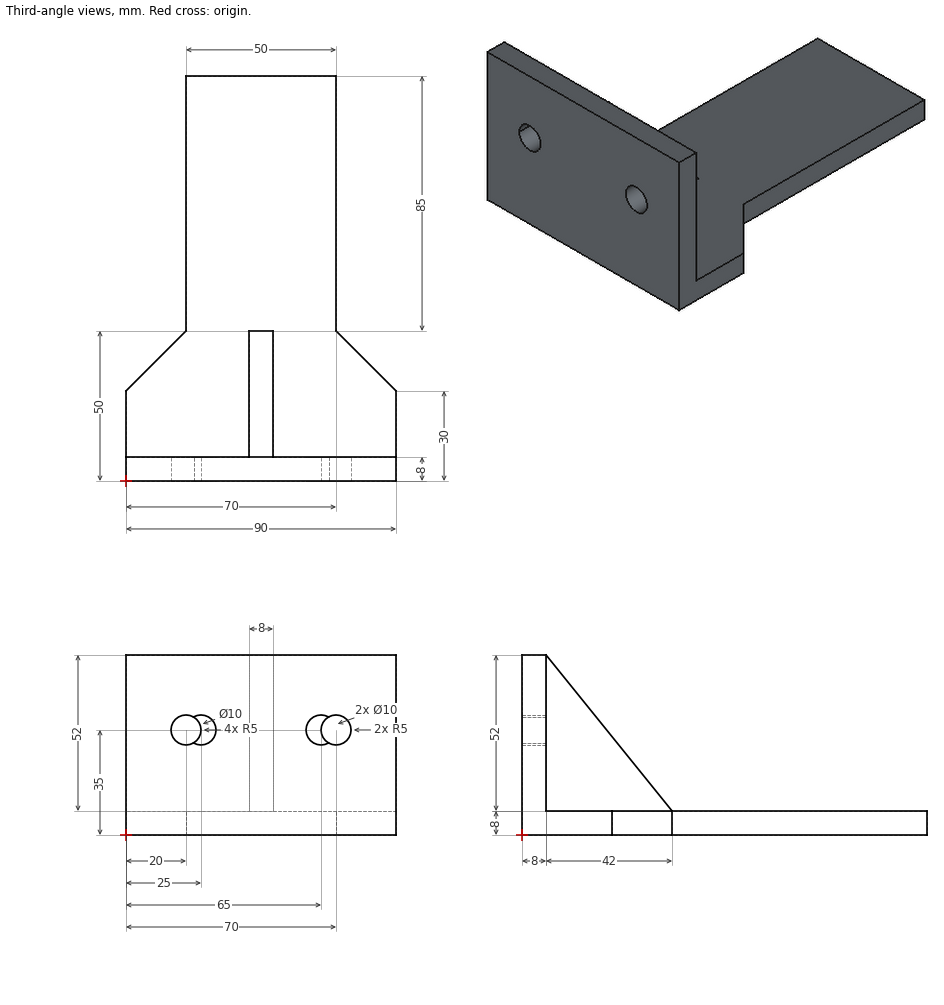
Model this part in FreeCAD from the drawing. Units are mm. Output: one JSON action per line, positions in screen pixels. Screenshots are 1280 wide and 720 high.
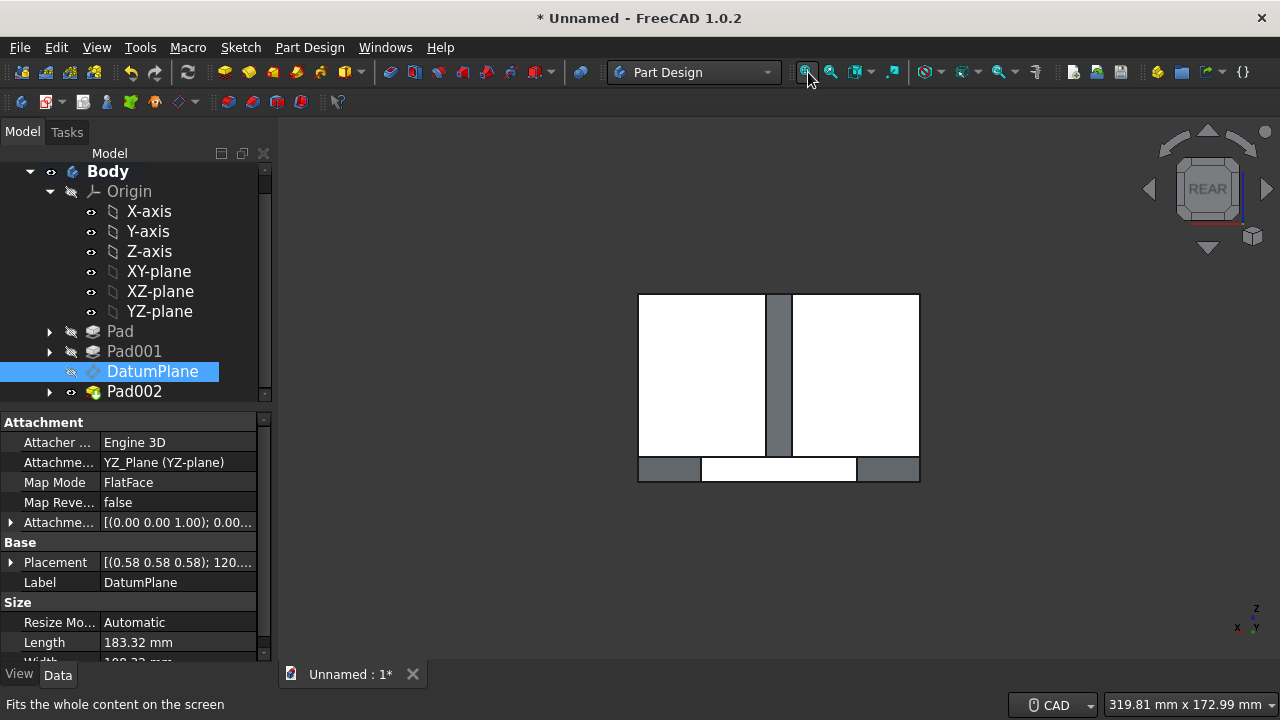
{"action": "left_click", "coordinate": [856, 374]}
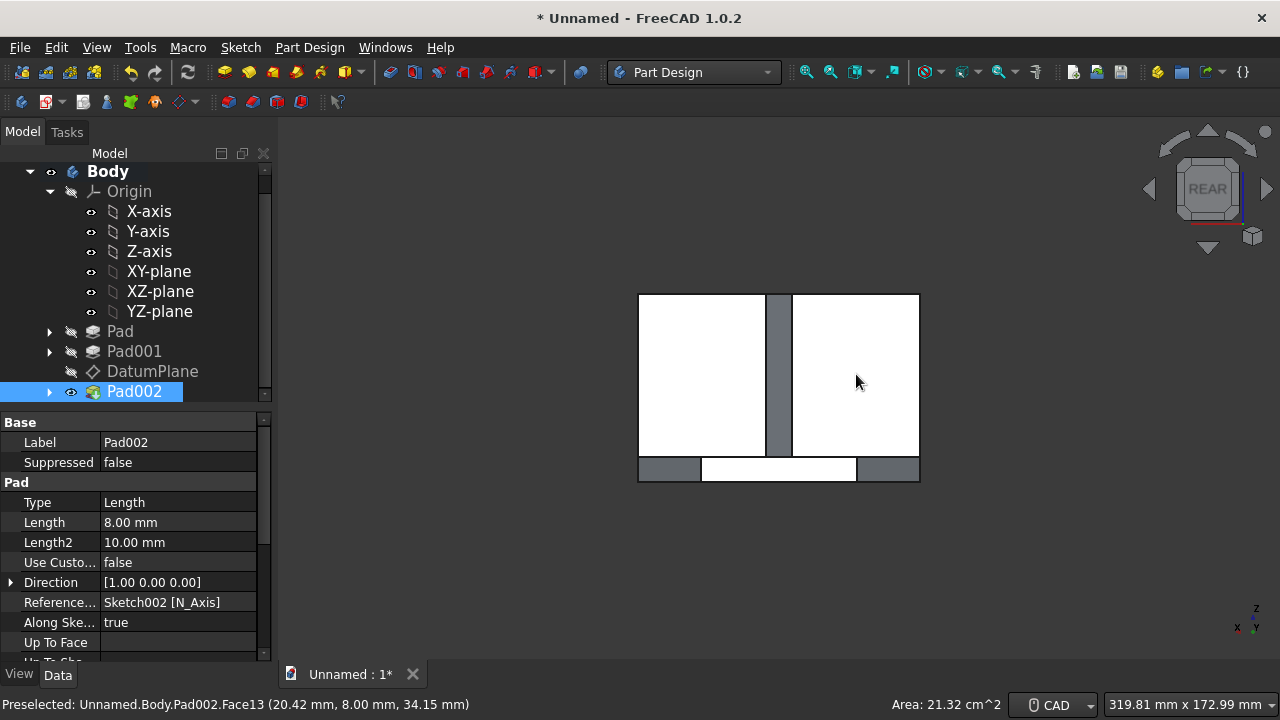
{"action": "left_click", "coordinate": [46, 102]}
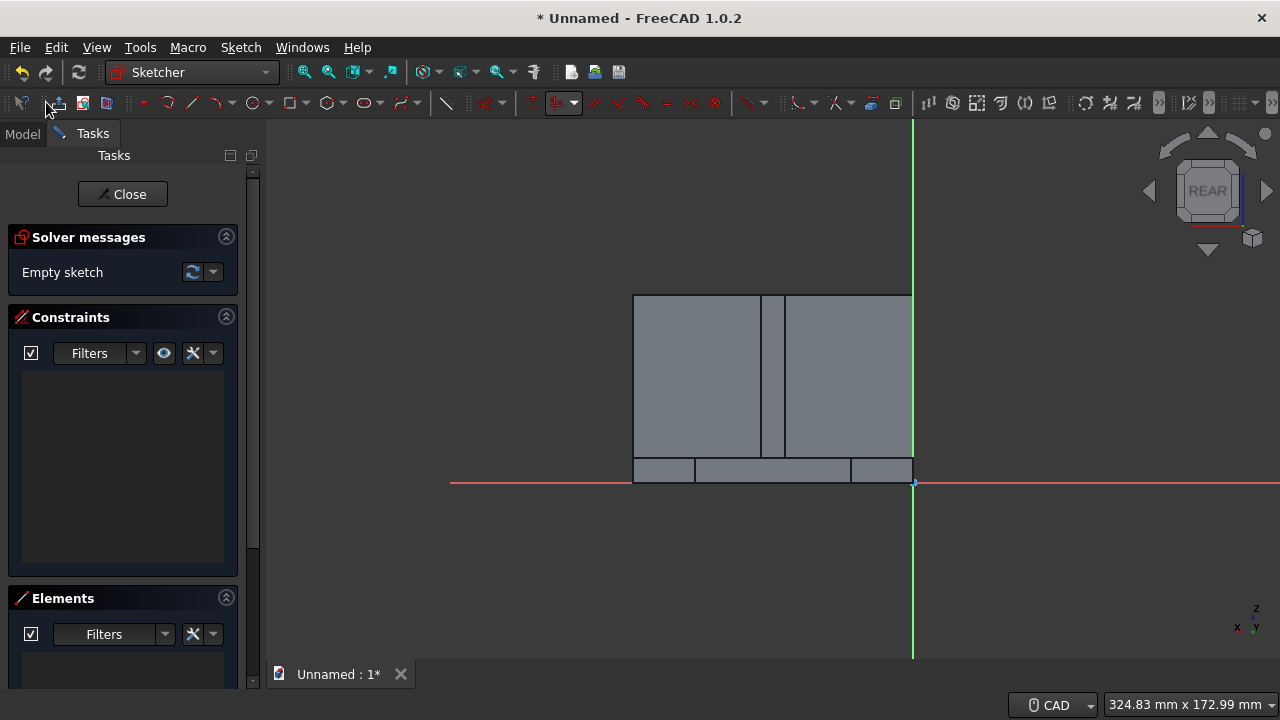
{"action": "scroll", "coordinate": [862, 438], "scroll_direction": "up", "scroll_amount": 5}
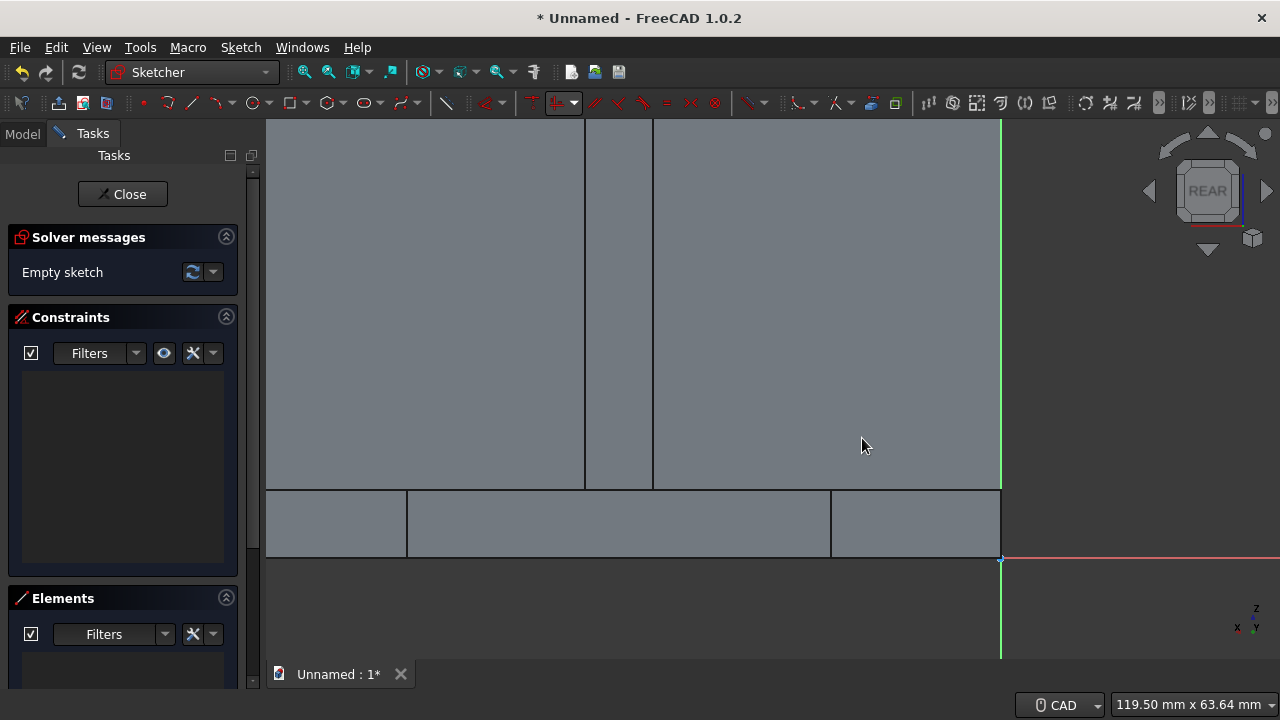
{"action": "left_click", "coordinate": [254, 104]}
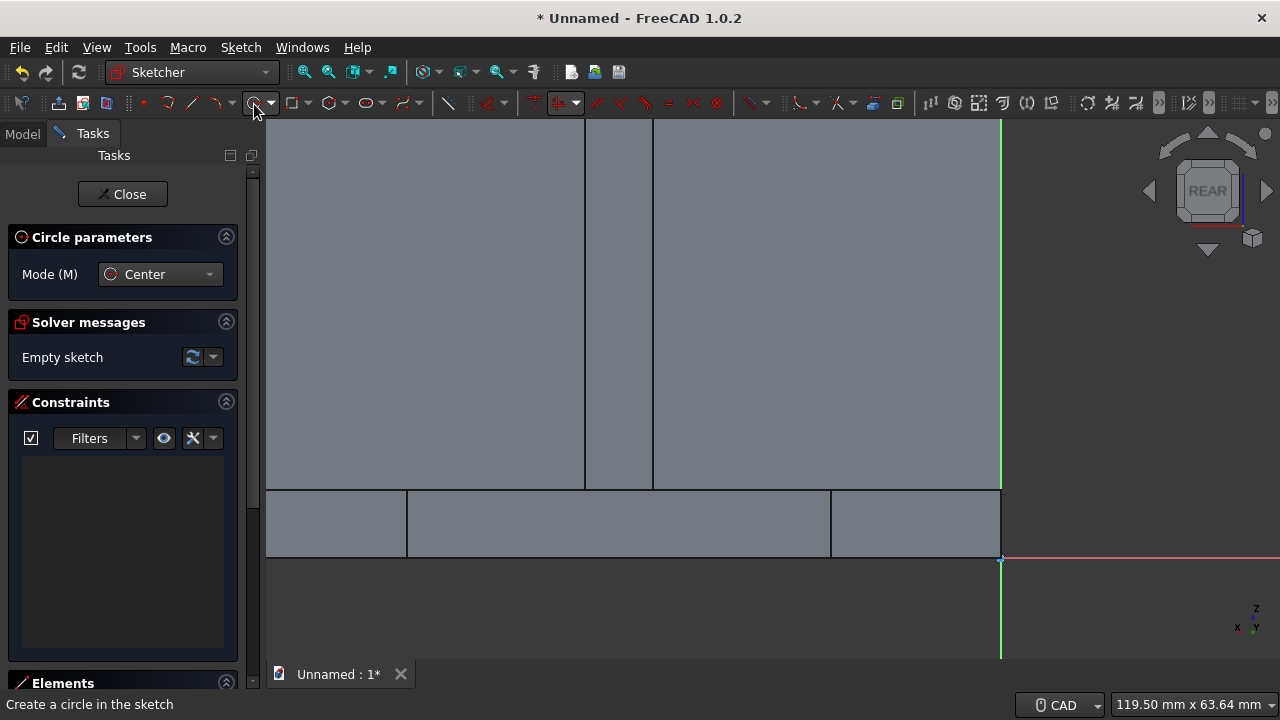
{"action": "left_click", "coordinate": [449, 261]}
{"action": "mouse_move", "coordinate": [479, 231]}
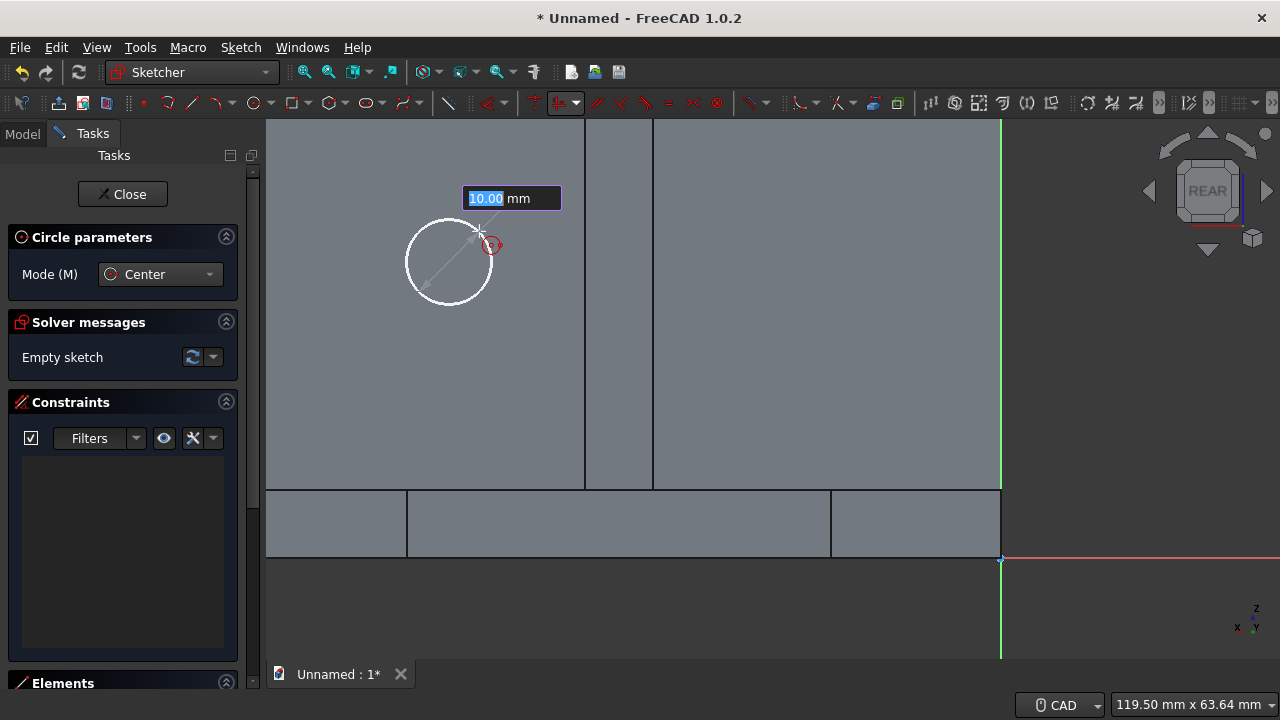
{"action": "type", "text": "10"}
{"action": "key", "text": "Return"}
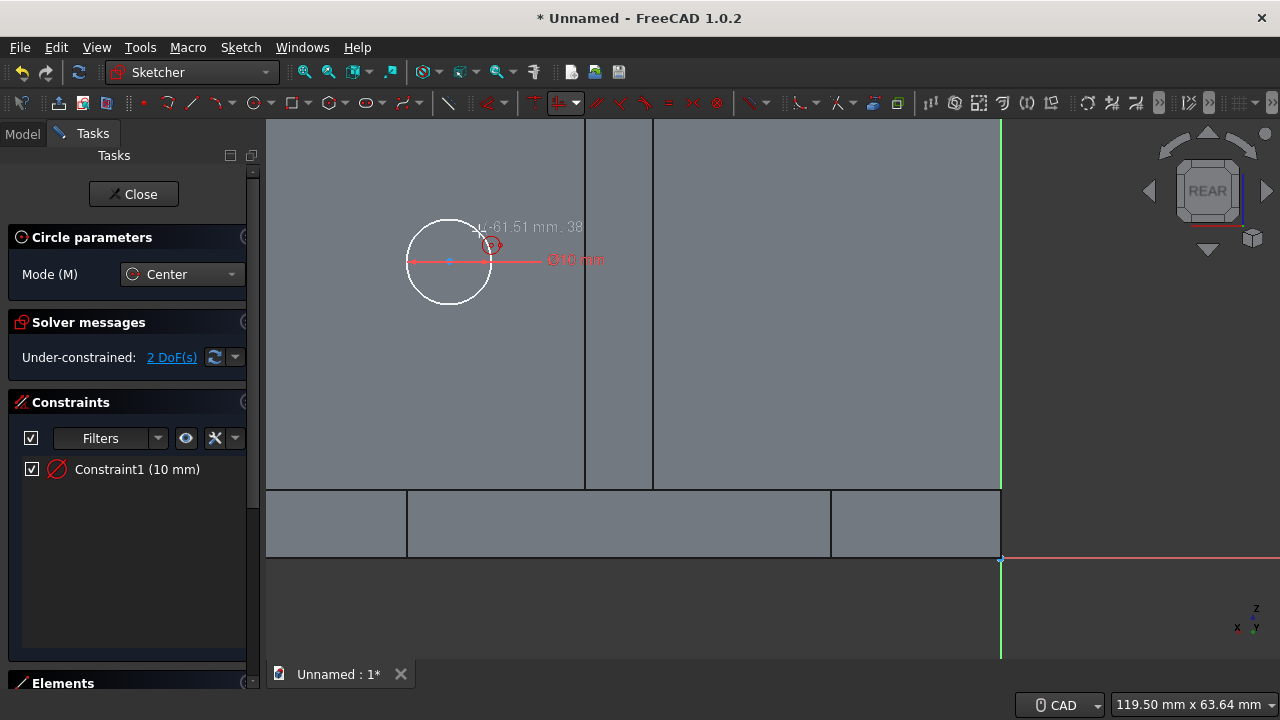
{"action": "left_click", "coordinate": [789, 261]}
{"action": "mouse_move", "coordinate": [819, 231]}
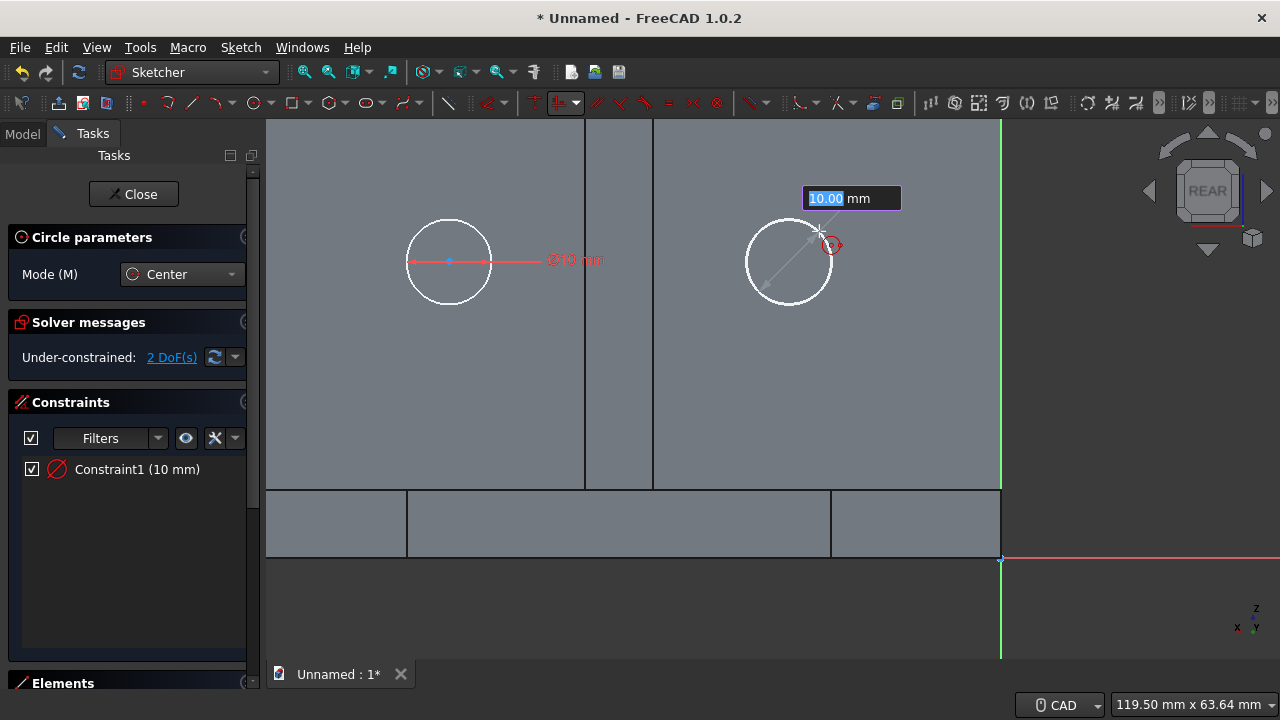
{"action": "type", "text": "10"}
{"action": "key", "text": "Return"}
{"action": "key", "text": "Escape"}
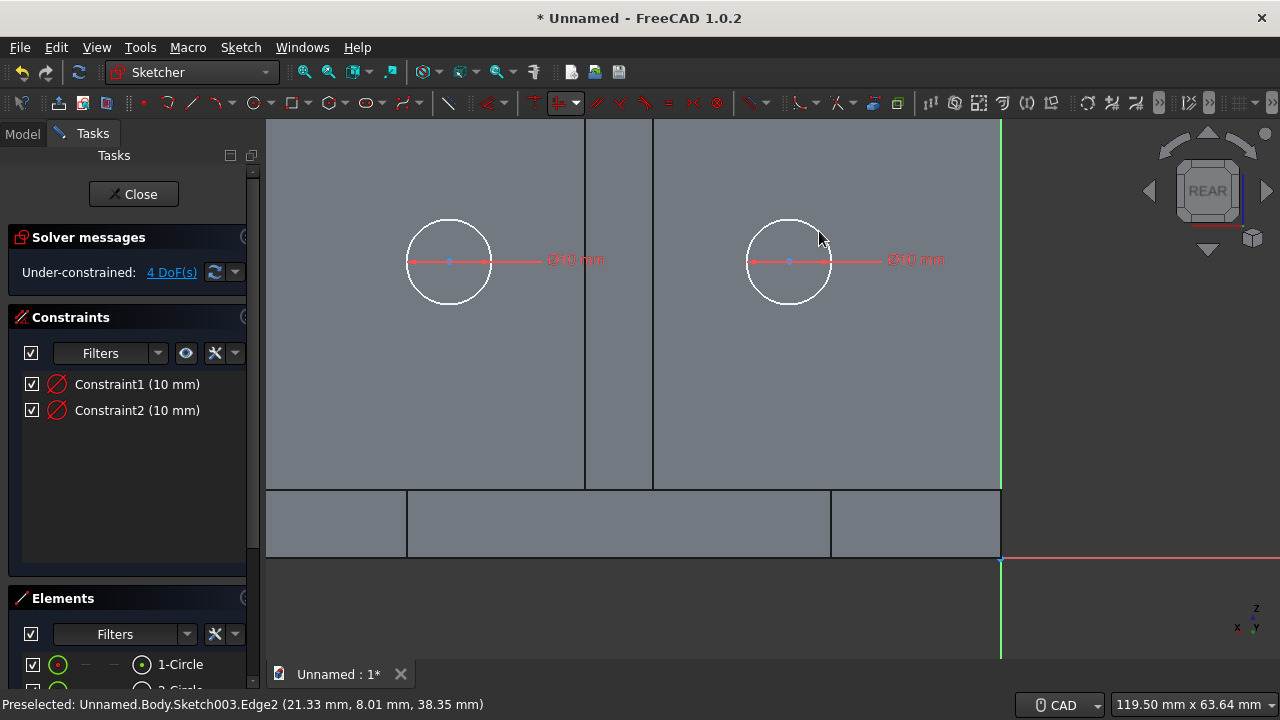
{"action": "left_click", "coordinate": [449, 262]}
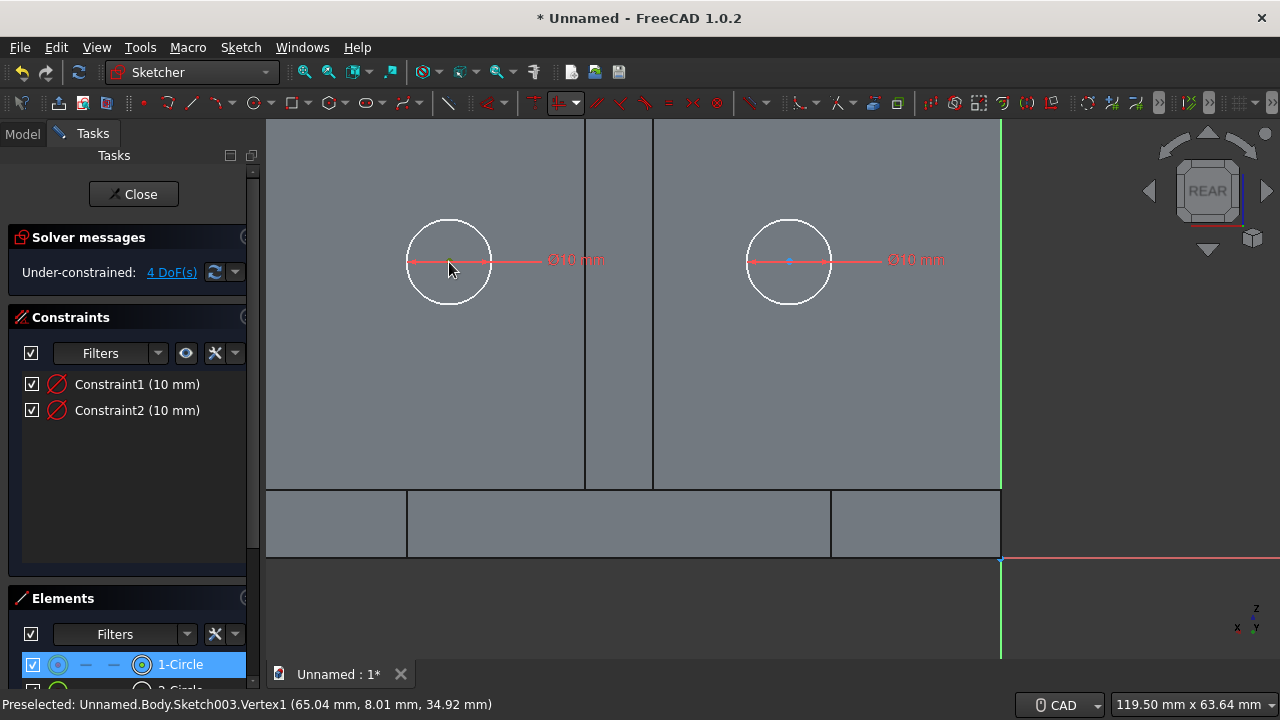
{"action": "left_click", "coordinate": [789, 262]}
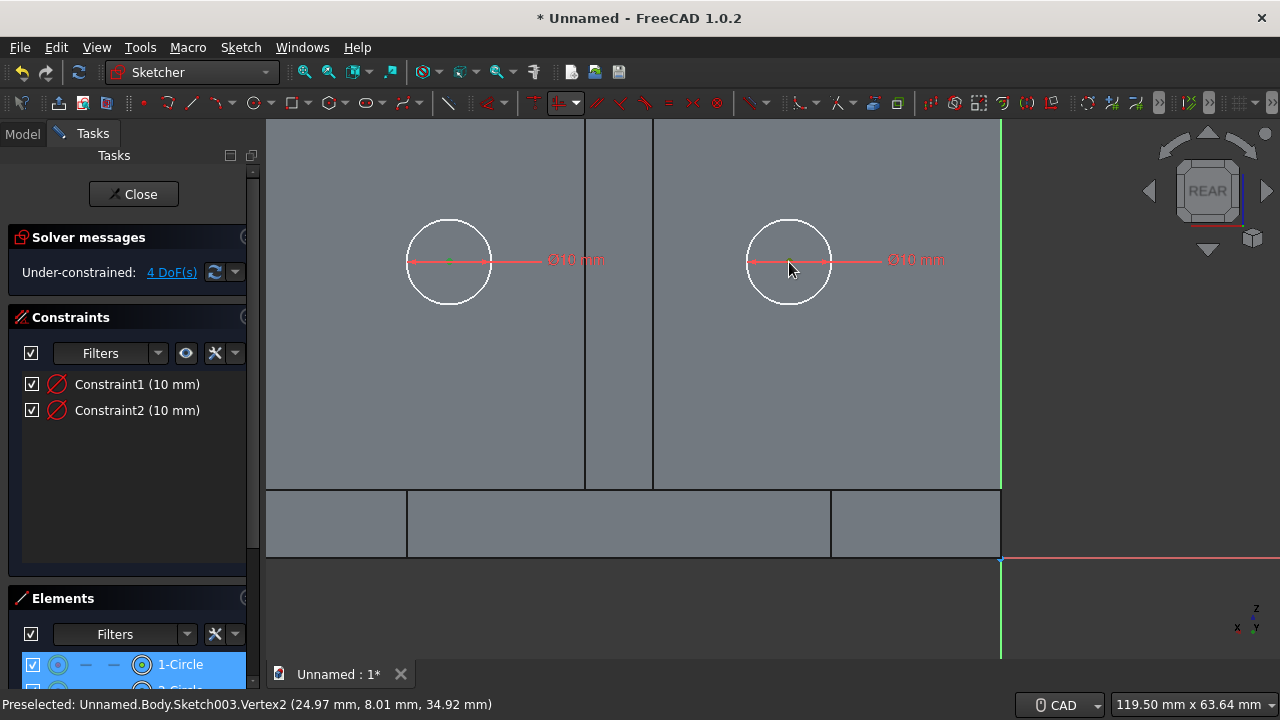
{"action": "left_click", "coordinate": [578, 104]}